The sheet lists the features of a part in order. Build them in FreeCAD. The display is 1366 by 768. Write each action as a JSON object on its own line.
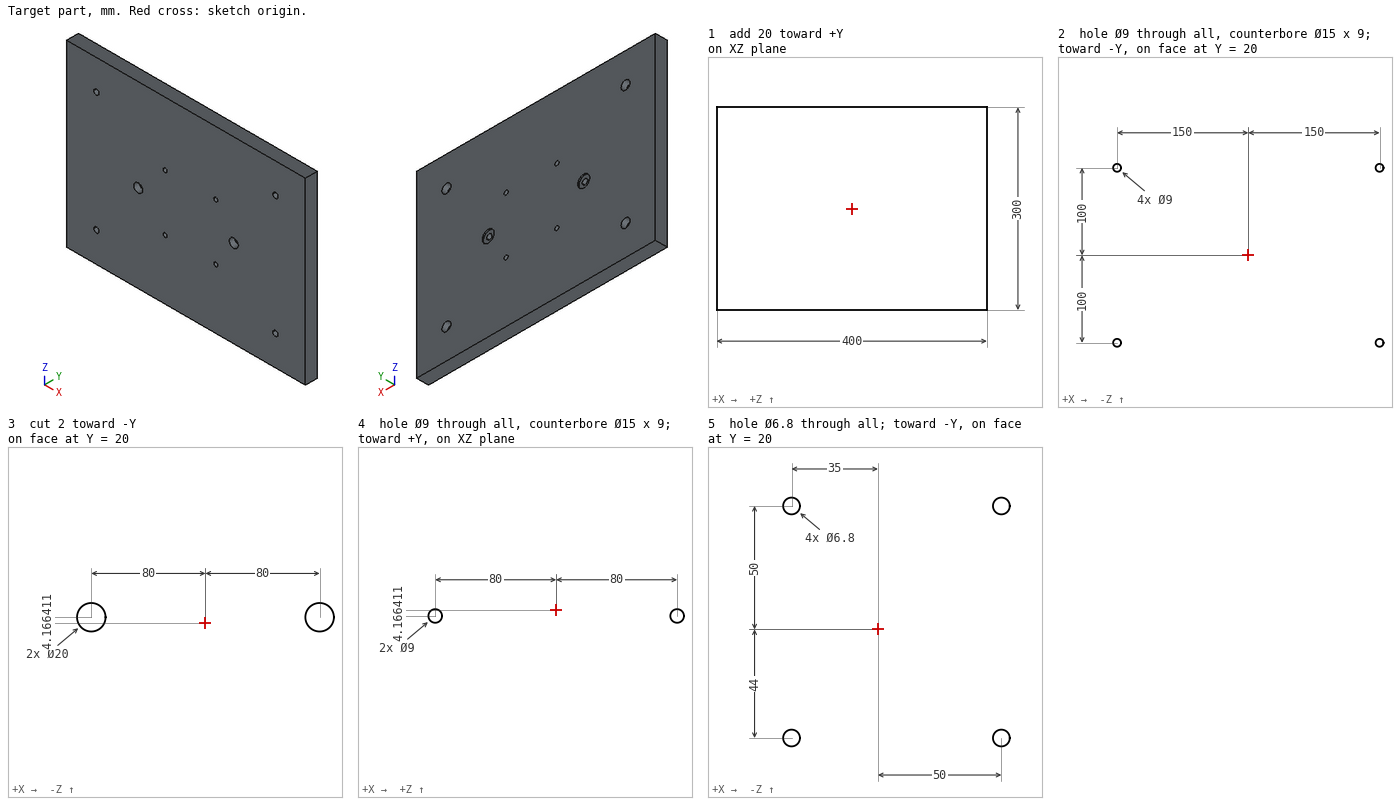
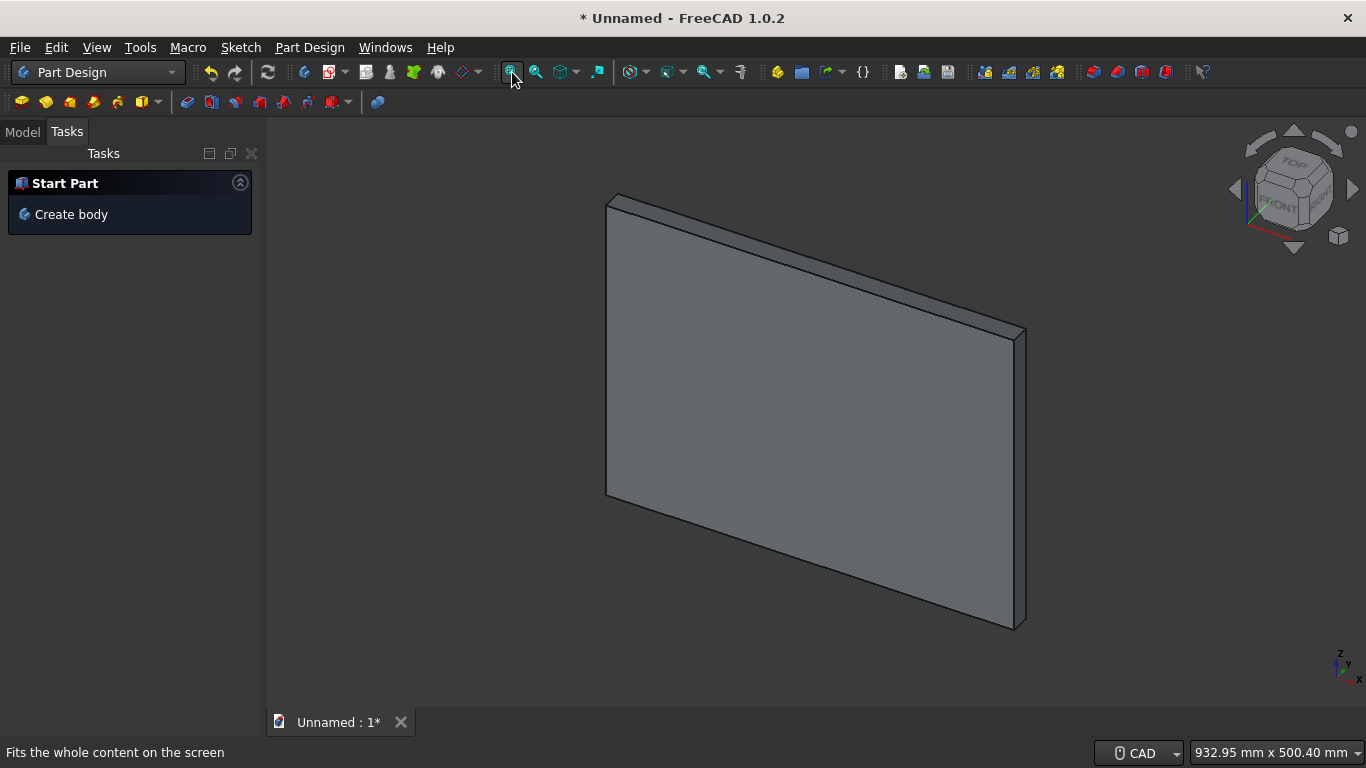
{"action": "key", "text": "4"}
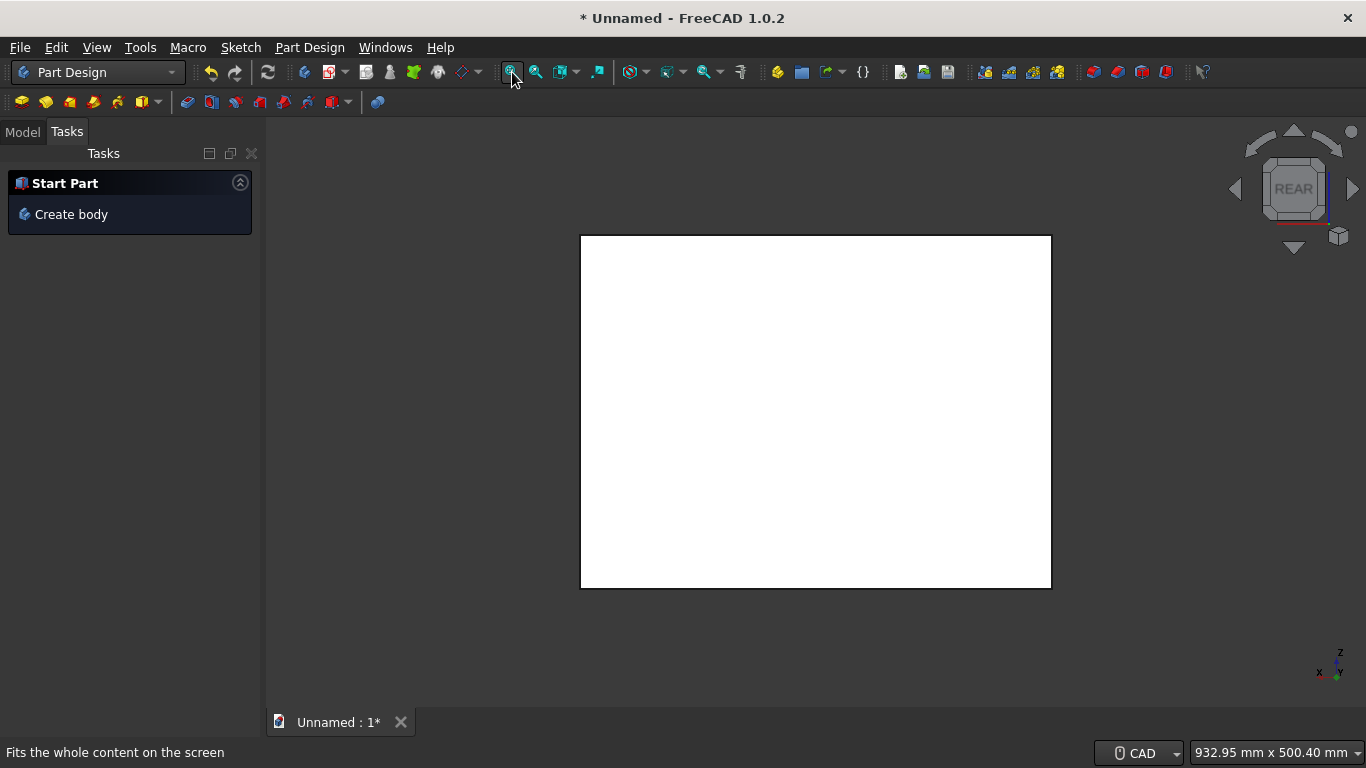
{"action": "left_click", "coordinate": [816, 411]}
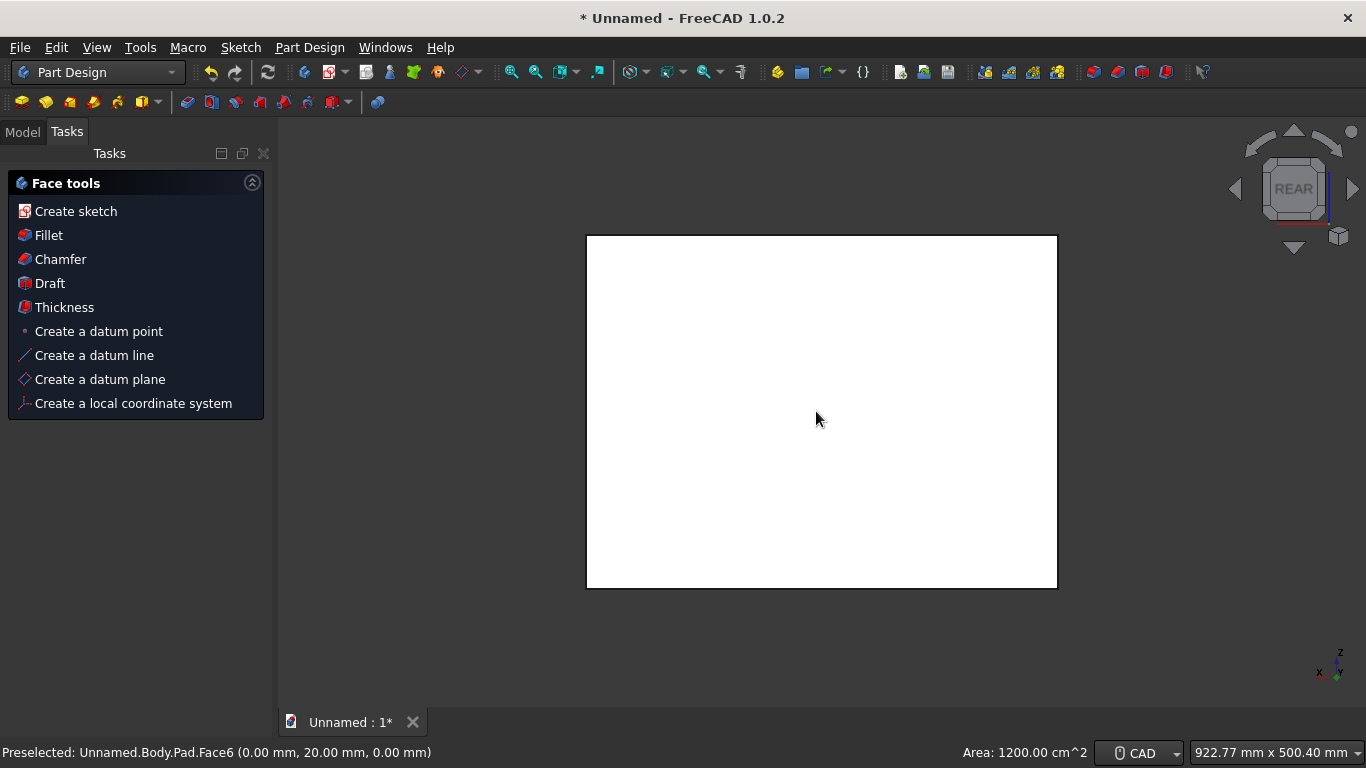
{"action": "left_click", "coordinate": [330, 72]}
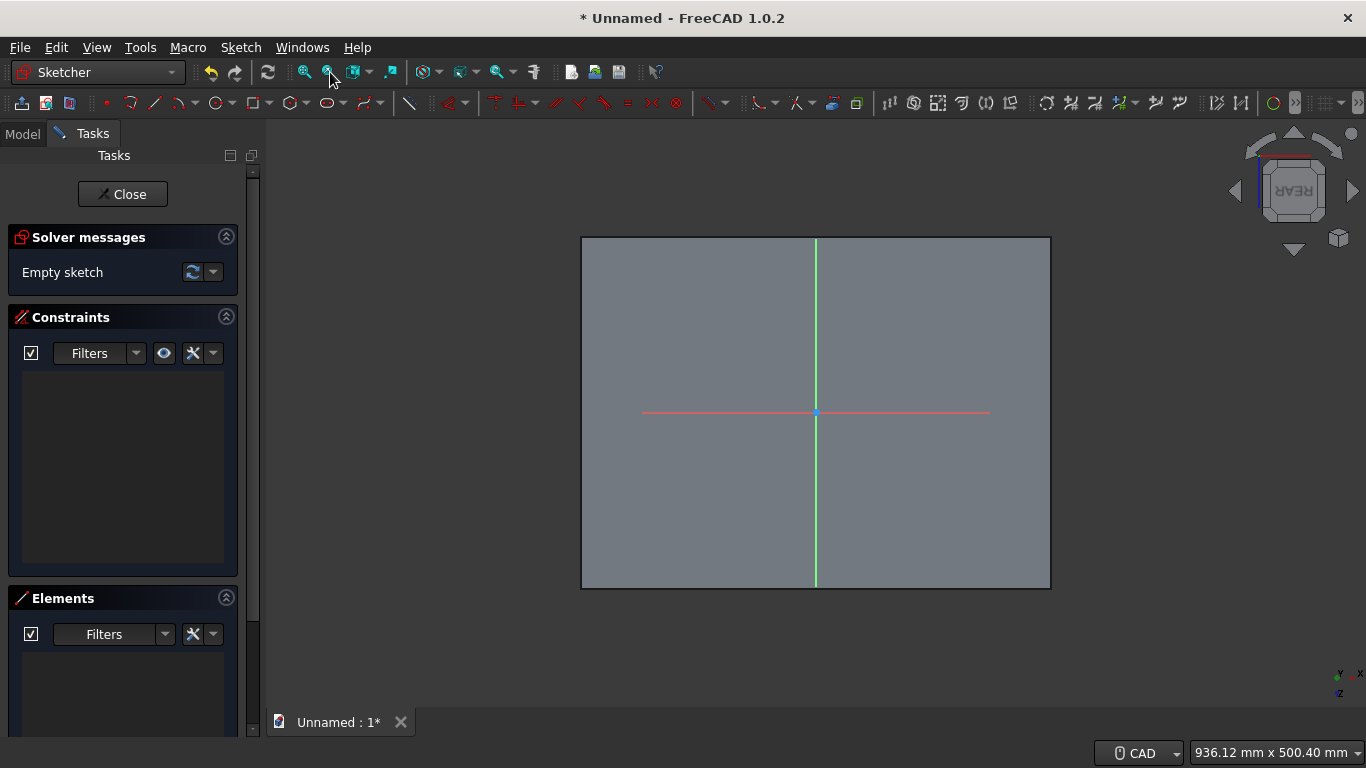
{"action": "scroll", "coordinate": [955, 413], "scroll_direction": "up", "scroll_amount": 2}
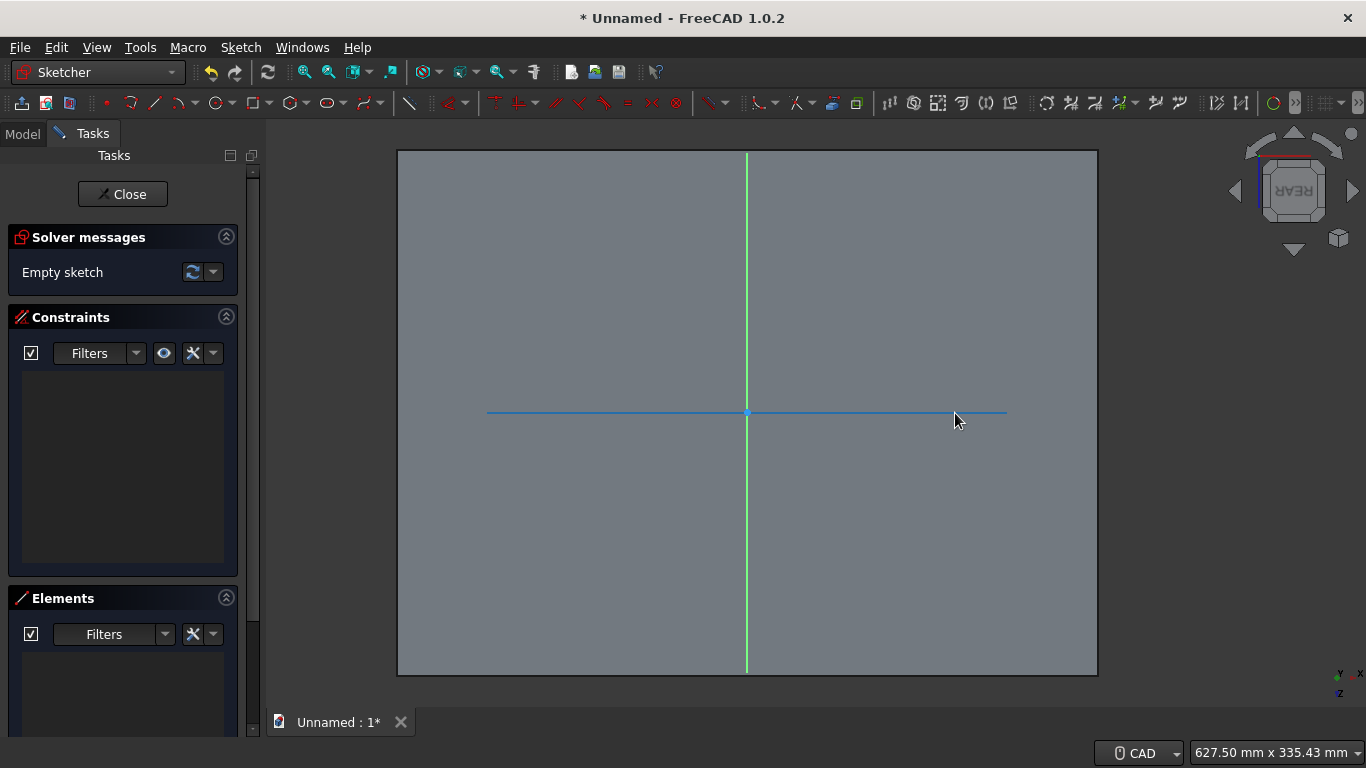
{"action": "left_click", "coordinate": [216, 104]}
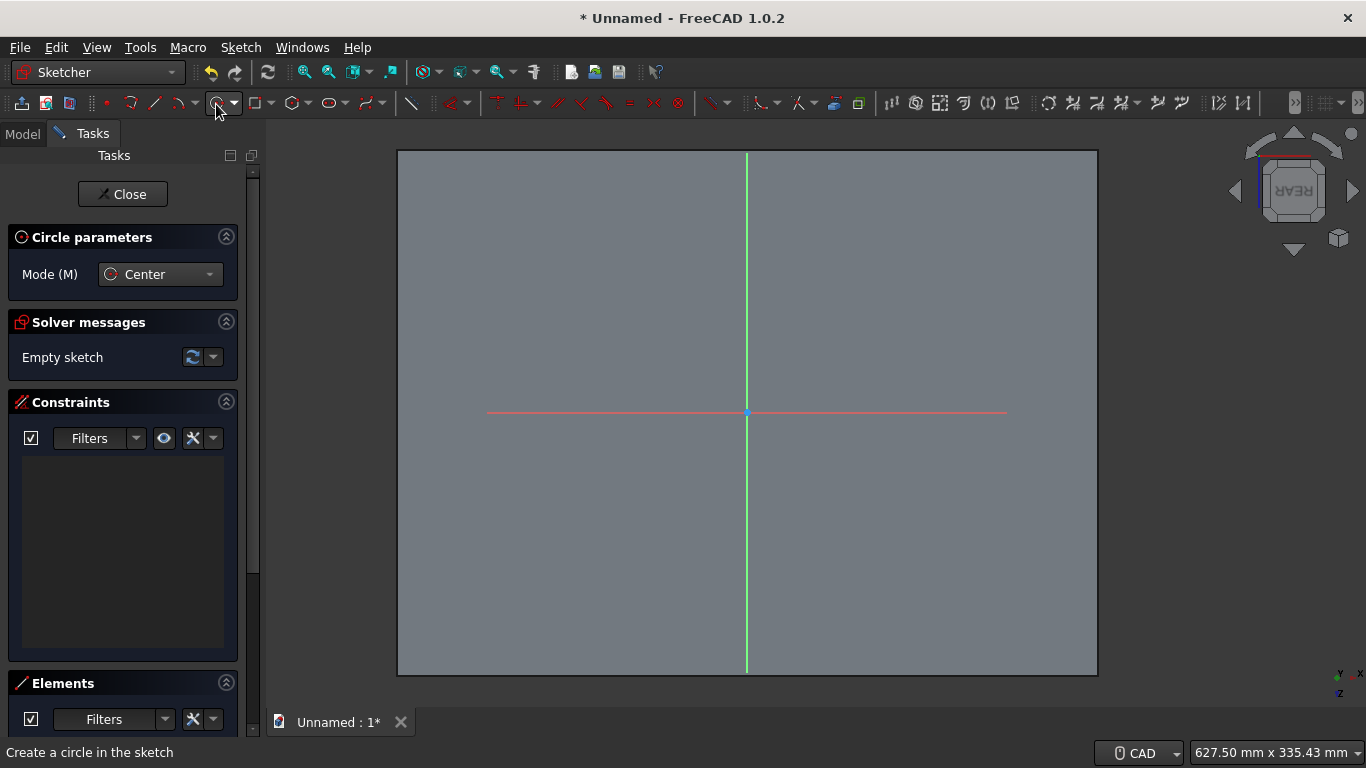
{"action": "scroll", "coordinate": [484, 237], "scroll_direction": "up", "scroll_amount": 6}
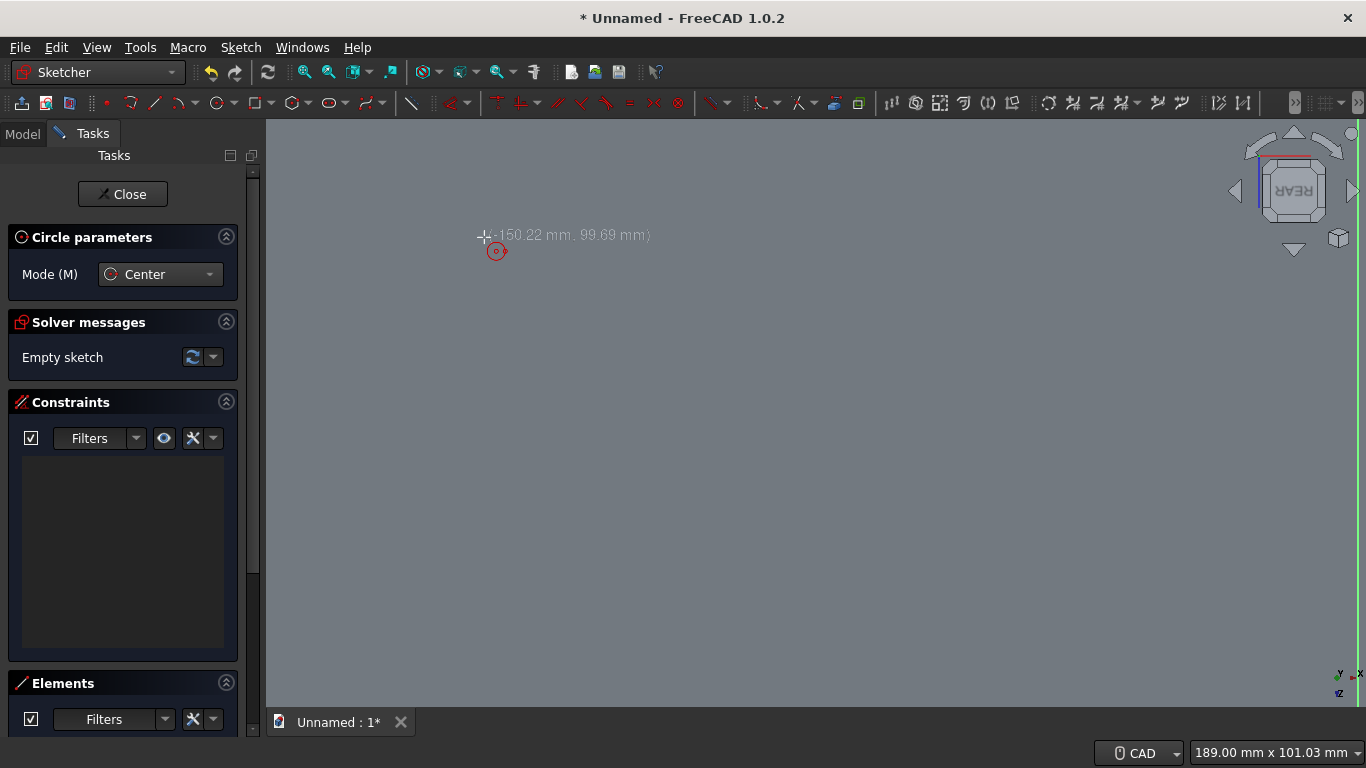
{"action": "left_click", "coordinate": [485, 238]}
{"action": "left_click", "coordinate": [503, 220]}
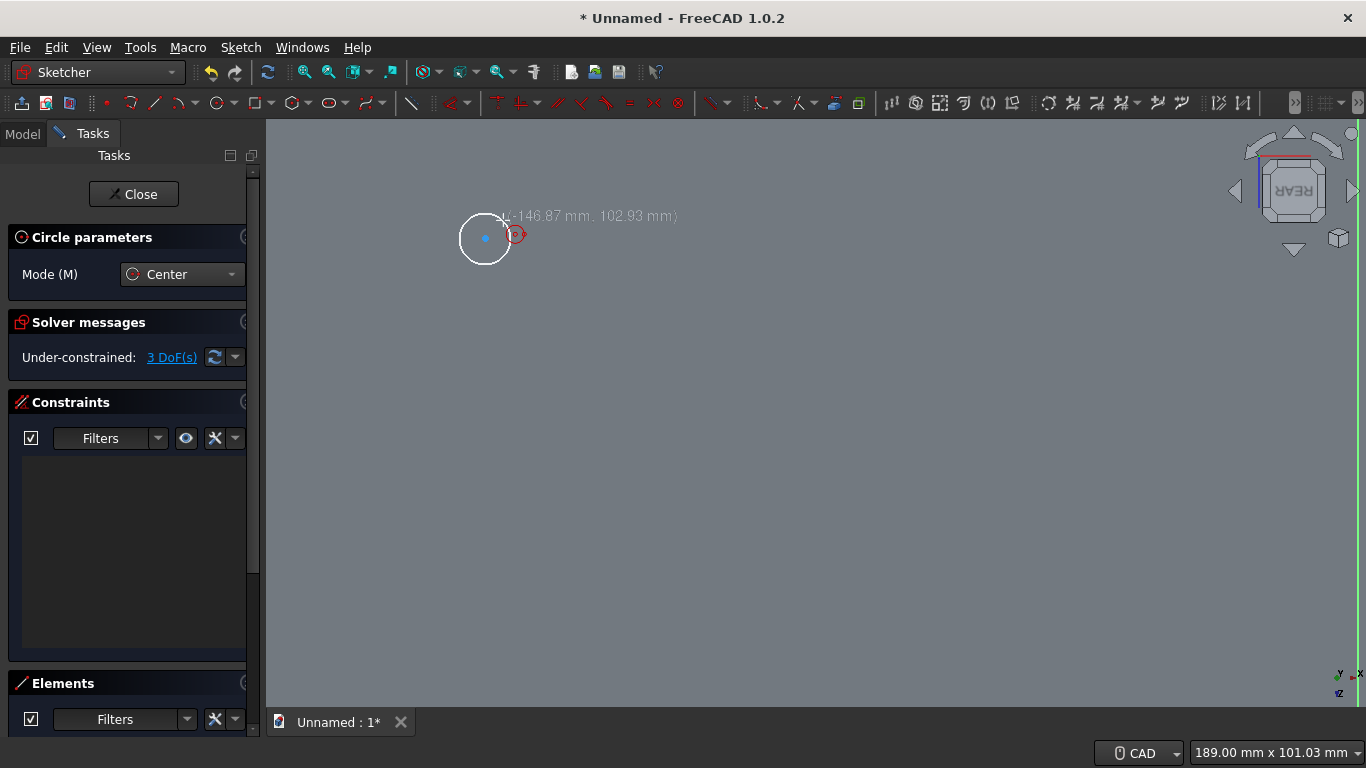
{"action": "scroll", "coordinate": [484, 238], "scroll_direction": "down", "scroll_amount": 6}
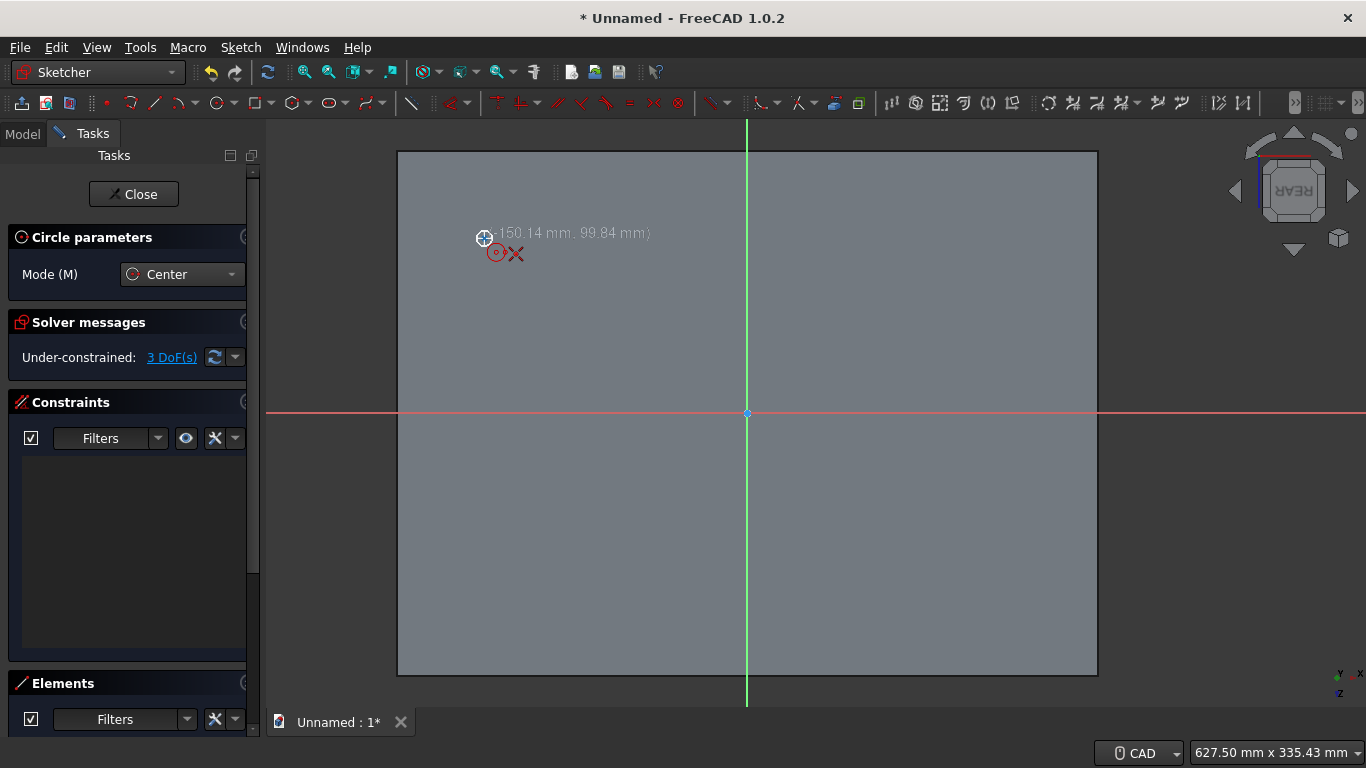
{"action": "scroll", "coordinate": [484, 589], "scroll_direction": "up", "scroll_amount": 6}